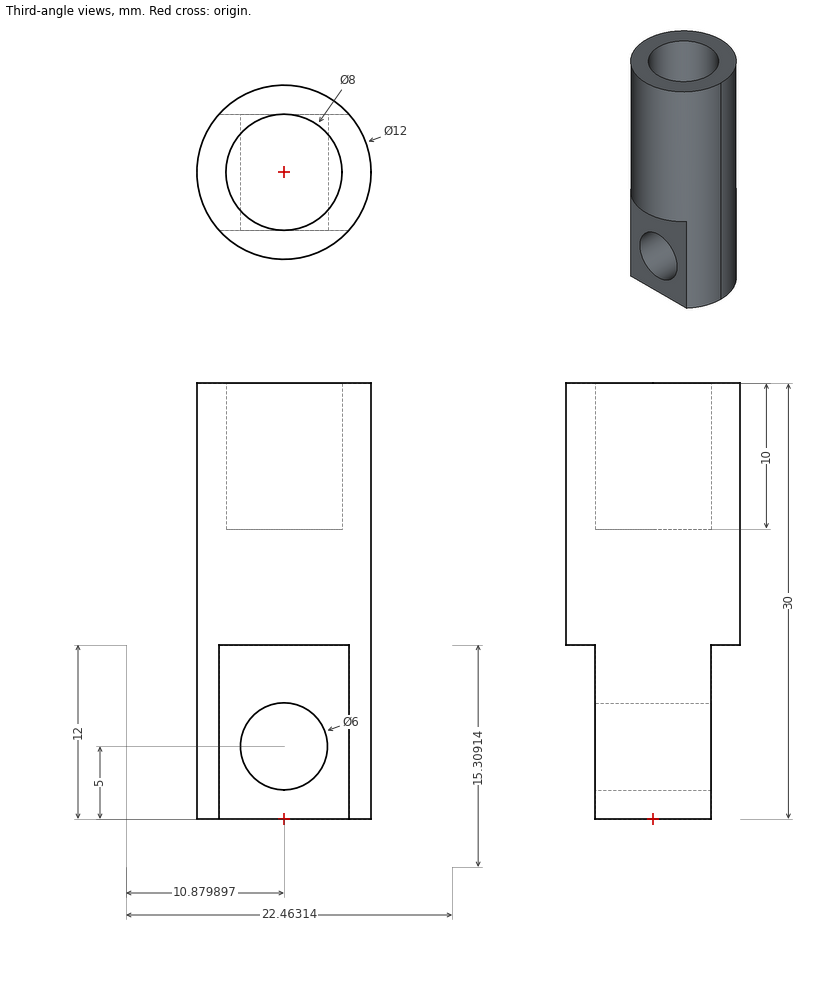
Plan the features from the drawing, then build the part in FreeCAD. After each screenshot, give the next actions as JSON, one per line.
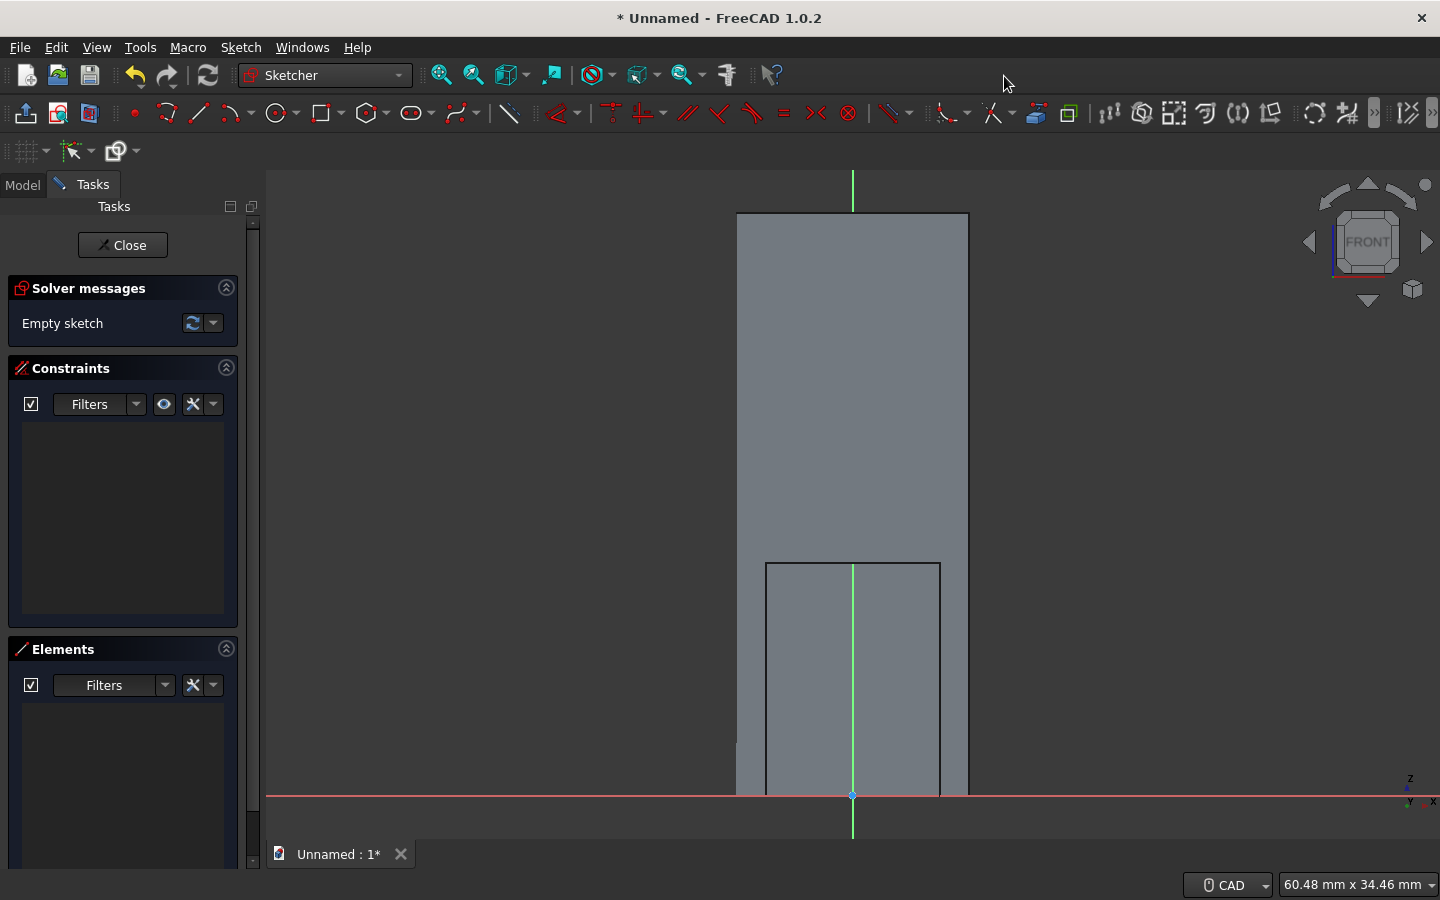
{"action": "scroll", "coordinate": [893, 811], "scroll_direction": "up", "scroll_amount": 5}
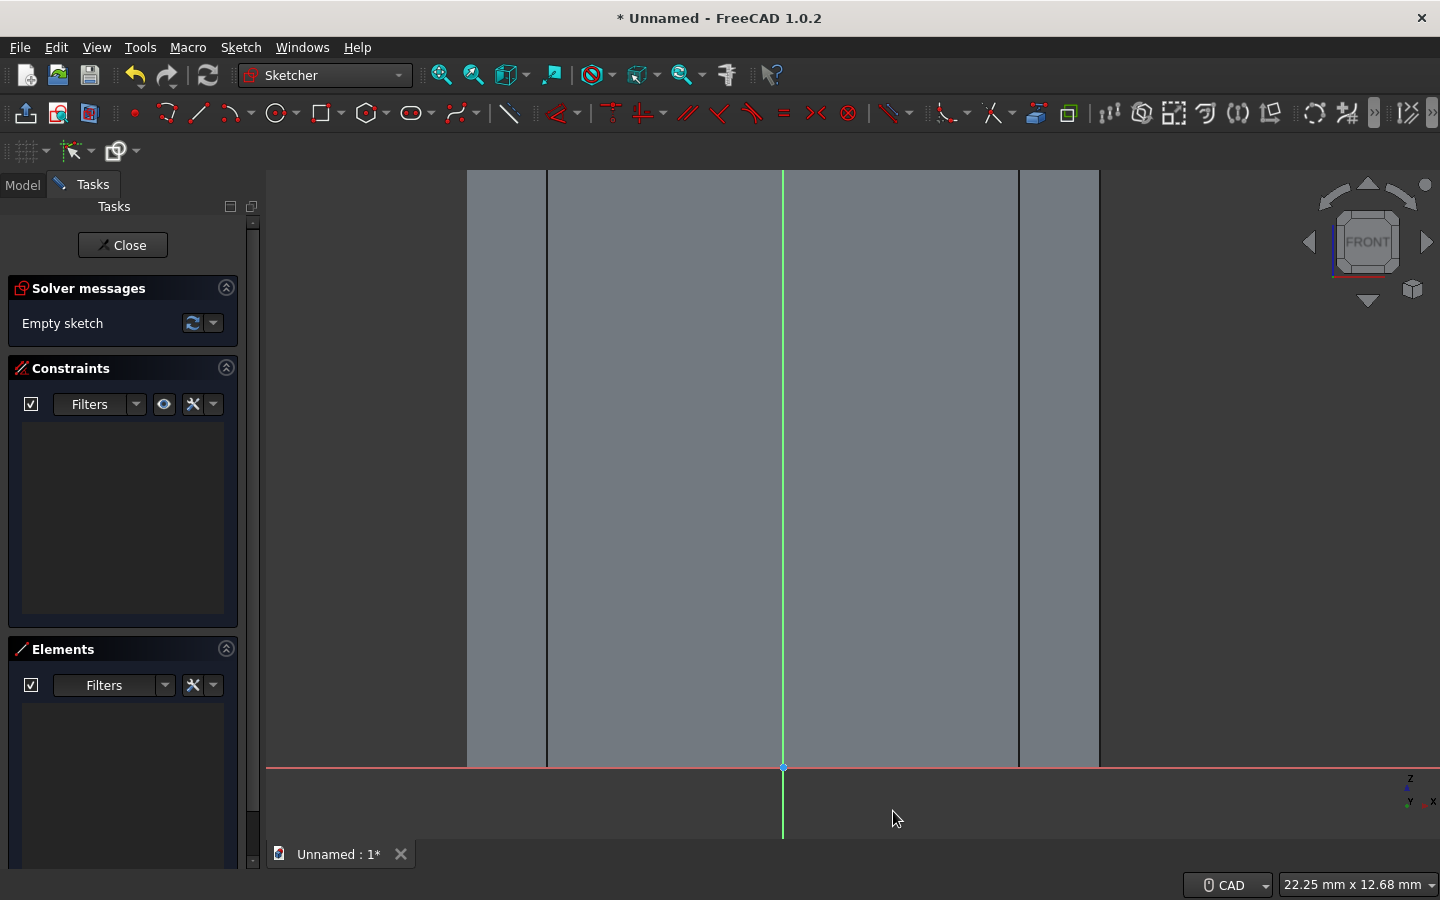
{"action": "left_click", "coordinate": [276, 114]}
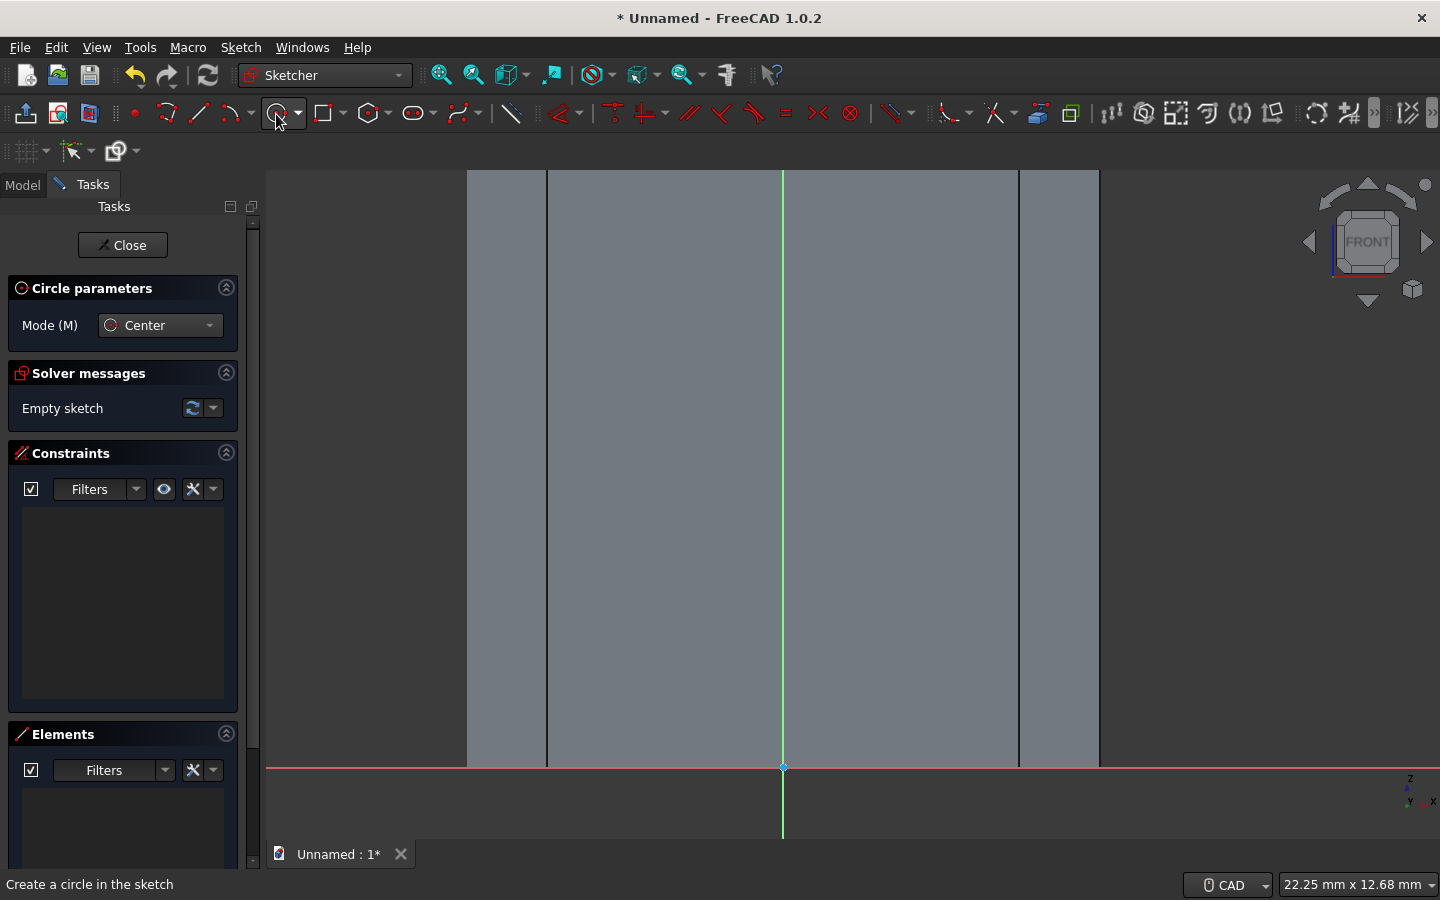
{"action": "left_click", "coordinate": [783, 504]}
{"action": "mouse_move", "coordinate": [895, 392]}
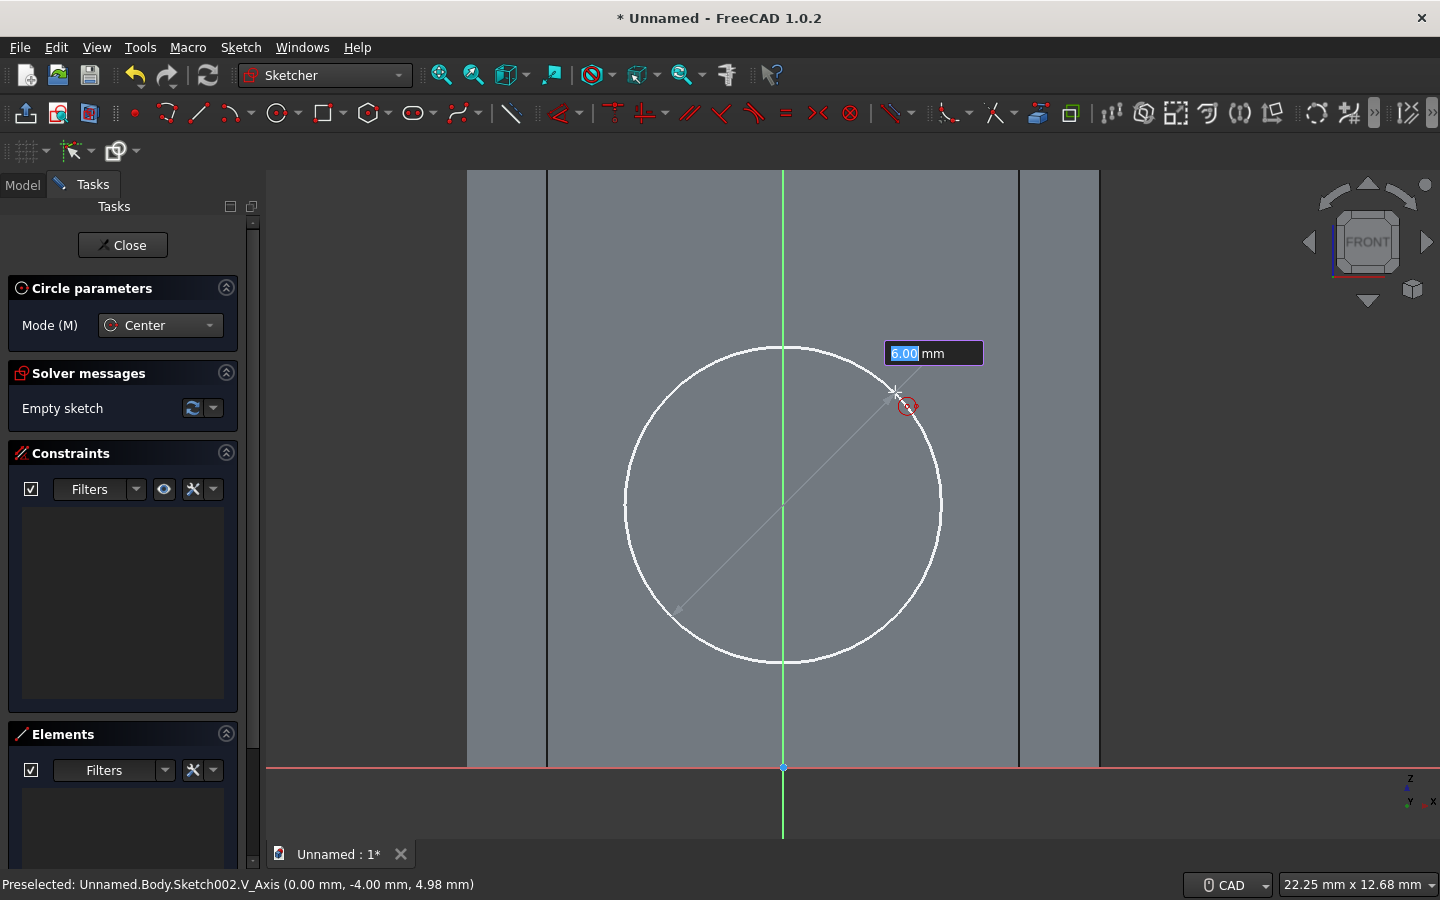
{"action": "type", "text": "6"}
{"action": "key", "text": "Return"}
{"action": "key", "text": "Escape"}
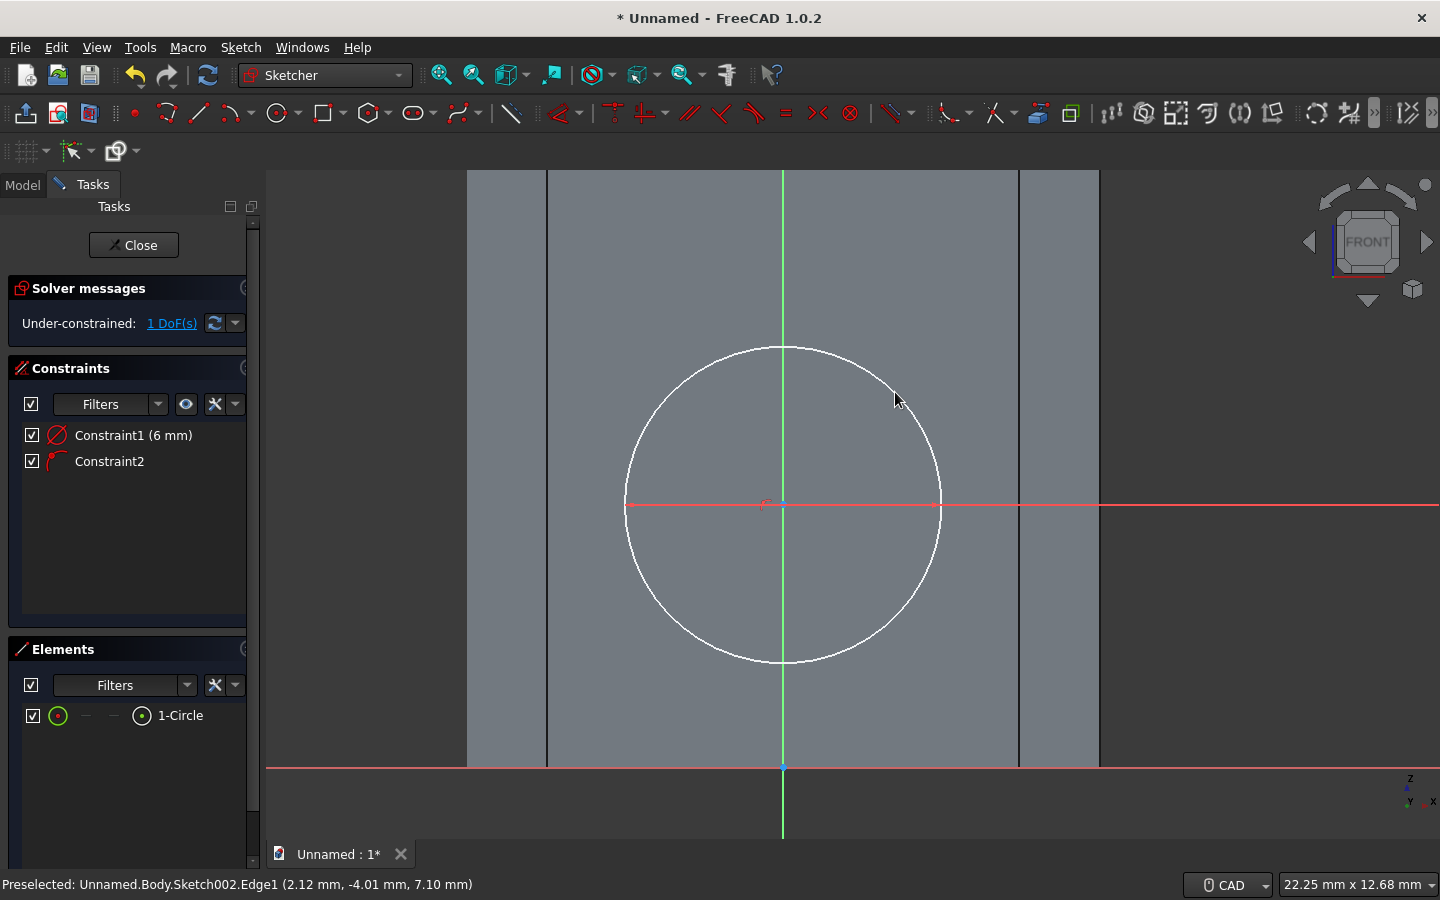
{"action": "left_click", "coordinate": [558, 114]}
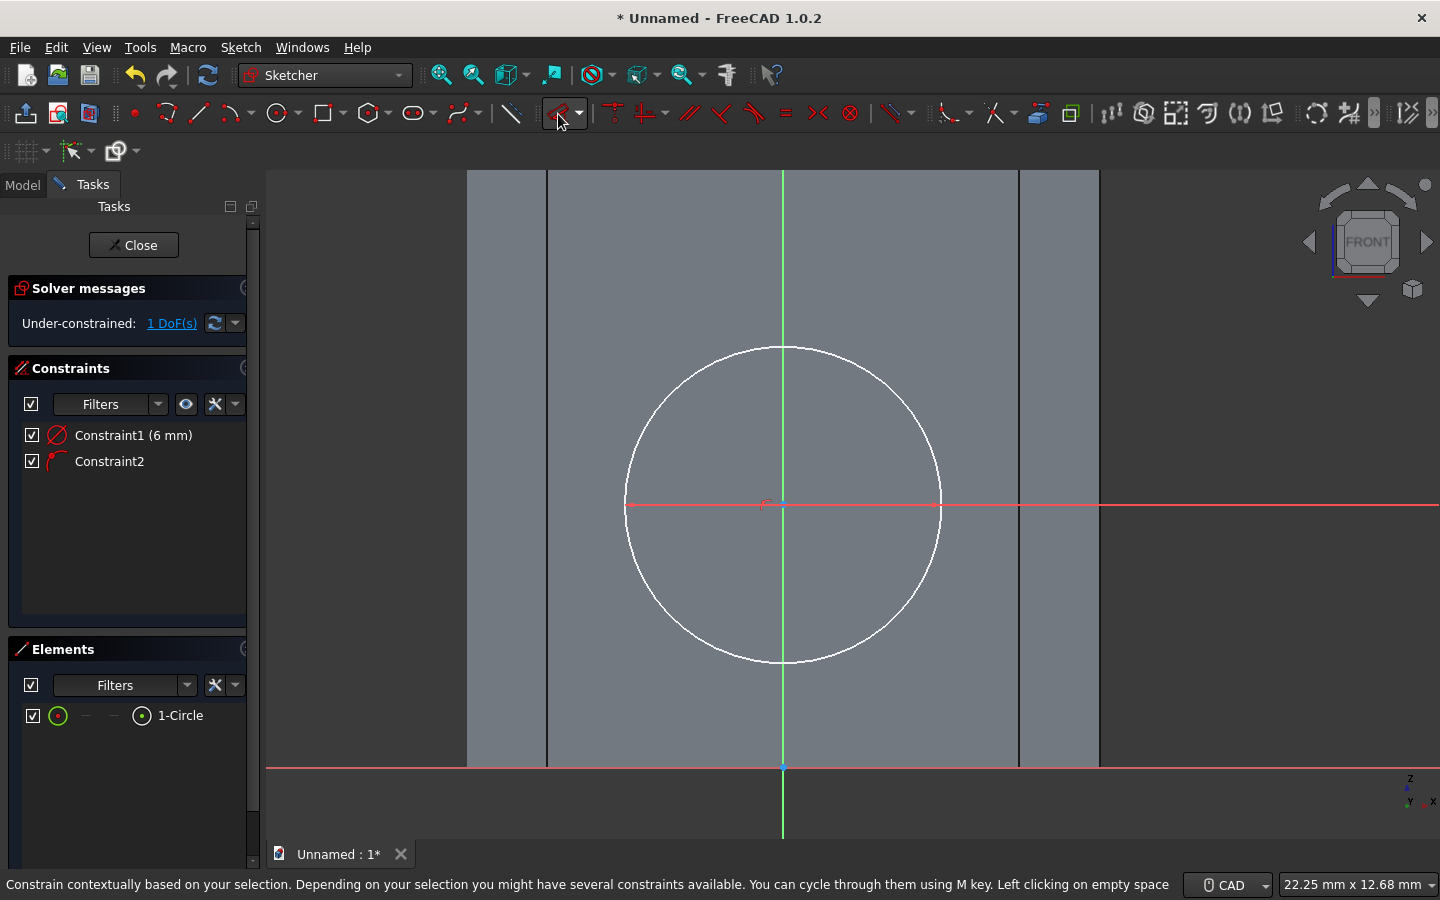
{"action": "left_click", "coordinate": [783, 505]}
{"action": "left_click", "coordinate": [817, 636]}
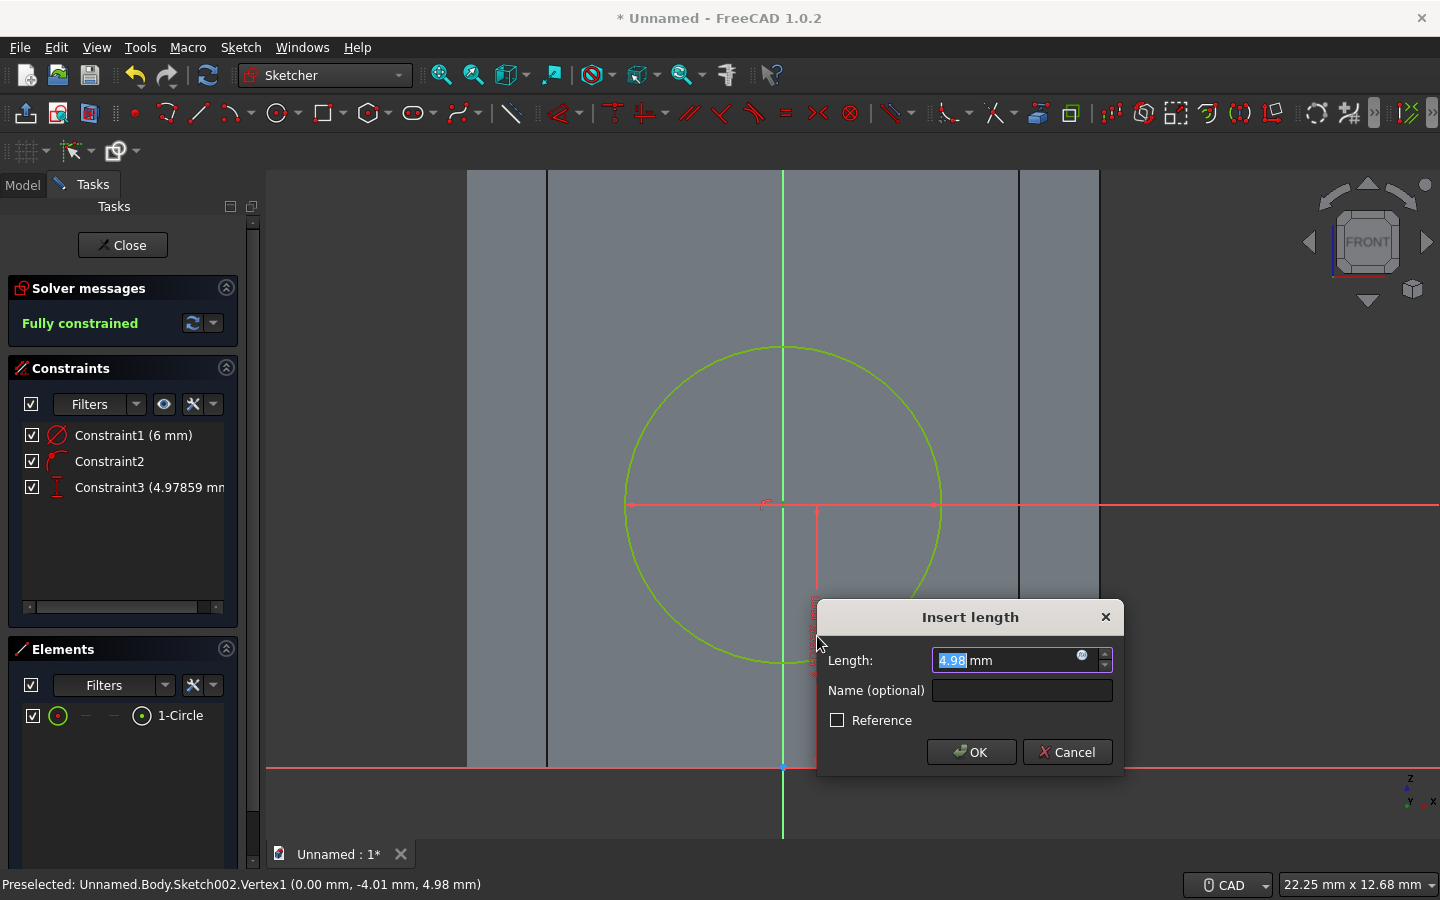
{"action": "type", "text": "5"}
{"action": "key", "text": "Return"}
{"action": "key", "text": "Escape"}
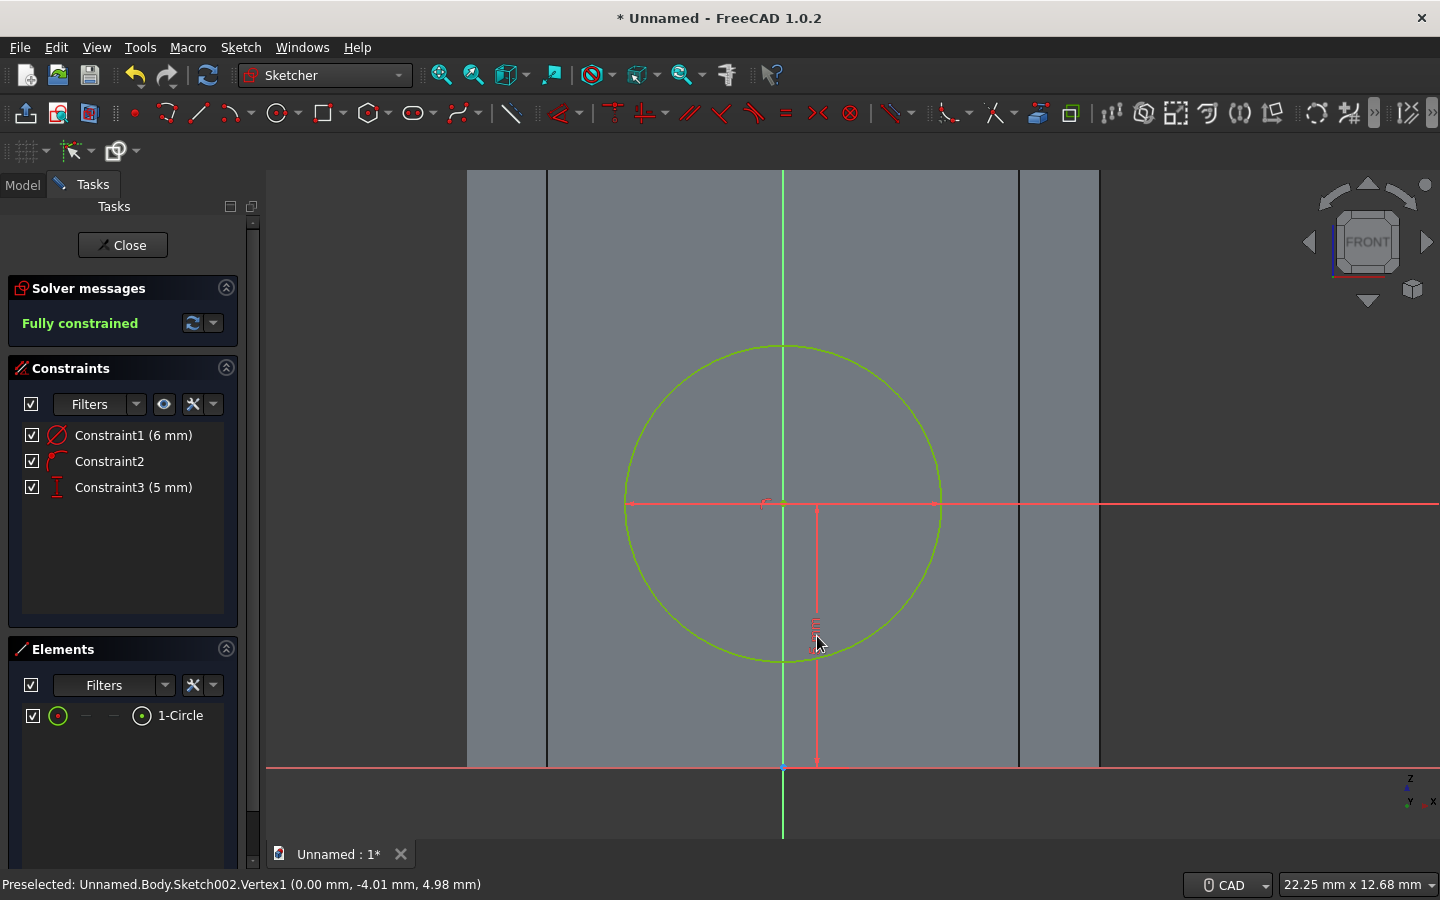
{"action": "left_click", "coordinate": [123, 245]}